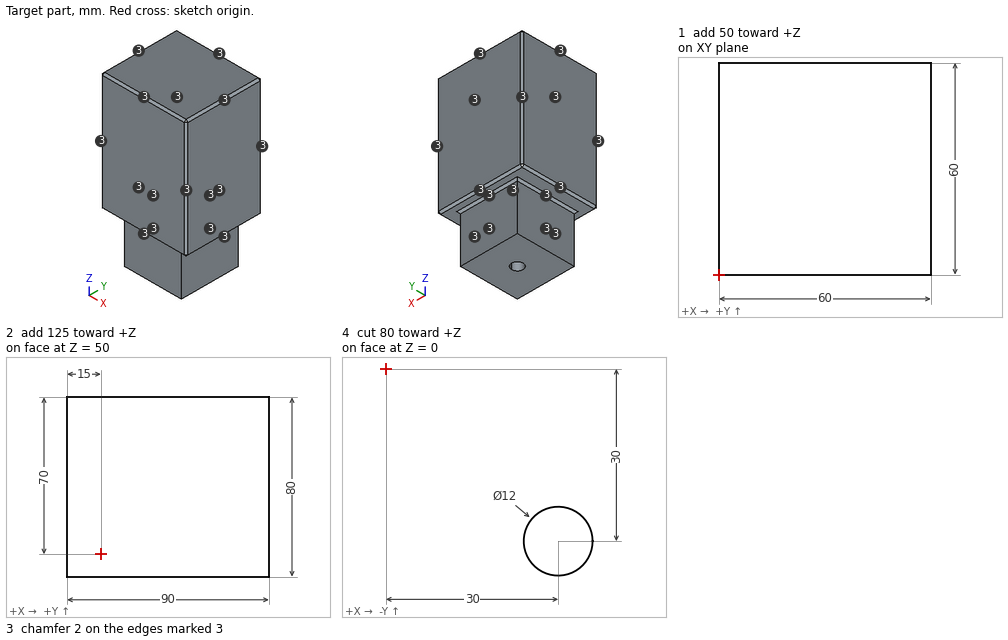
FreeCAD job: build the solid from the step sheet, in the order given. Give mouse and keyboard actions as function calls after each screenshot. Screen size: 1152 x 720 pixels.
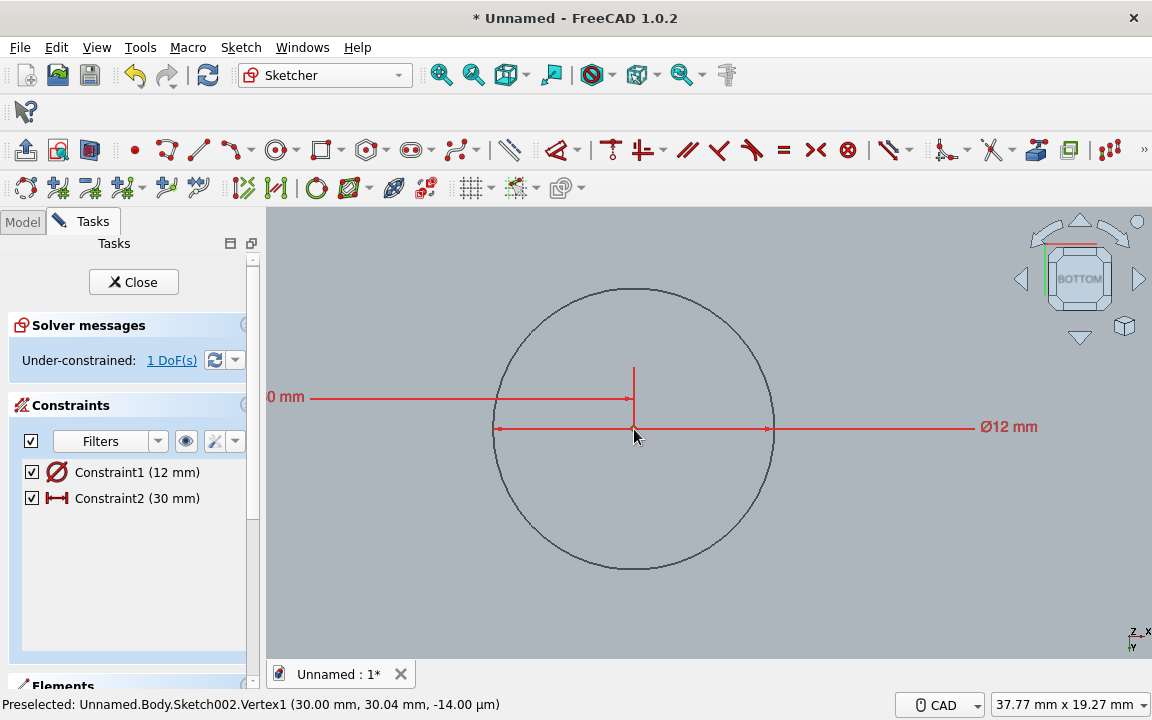
key(i)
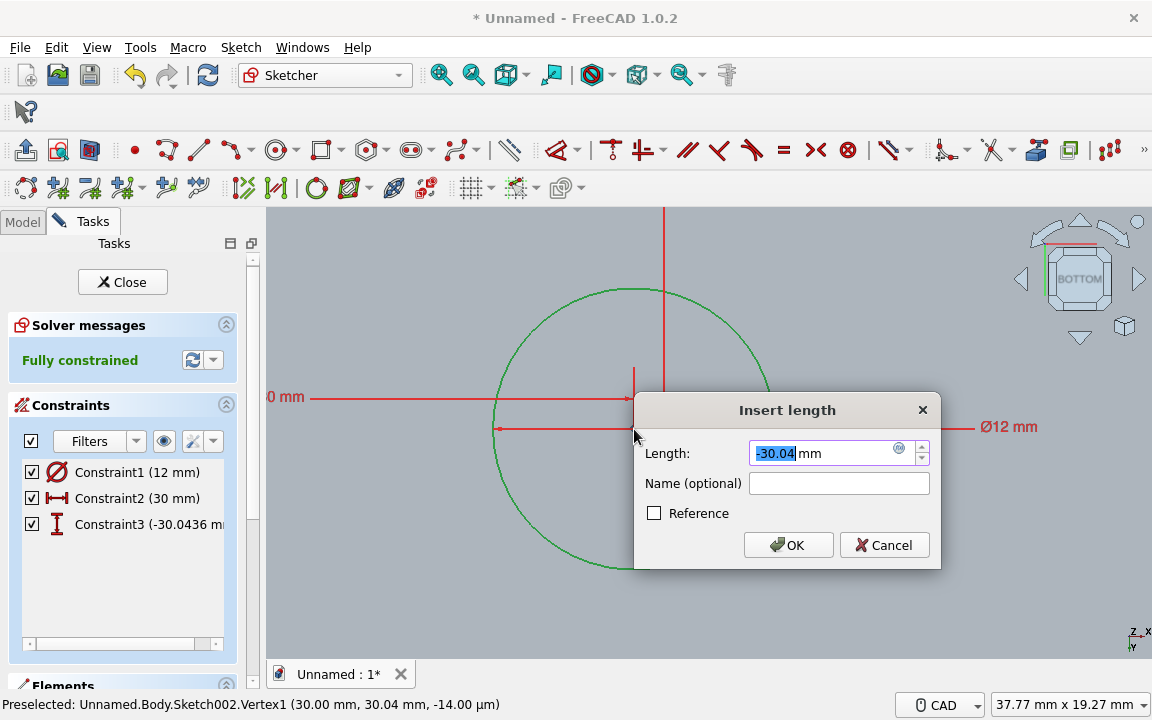
text(-30)
key(Return)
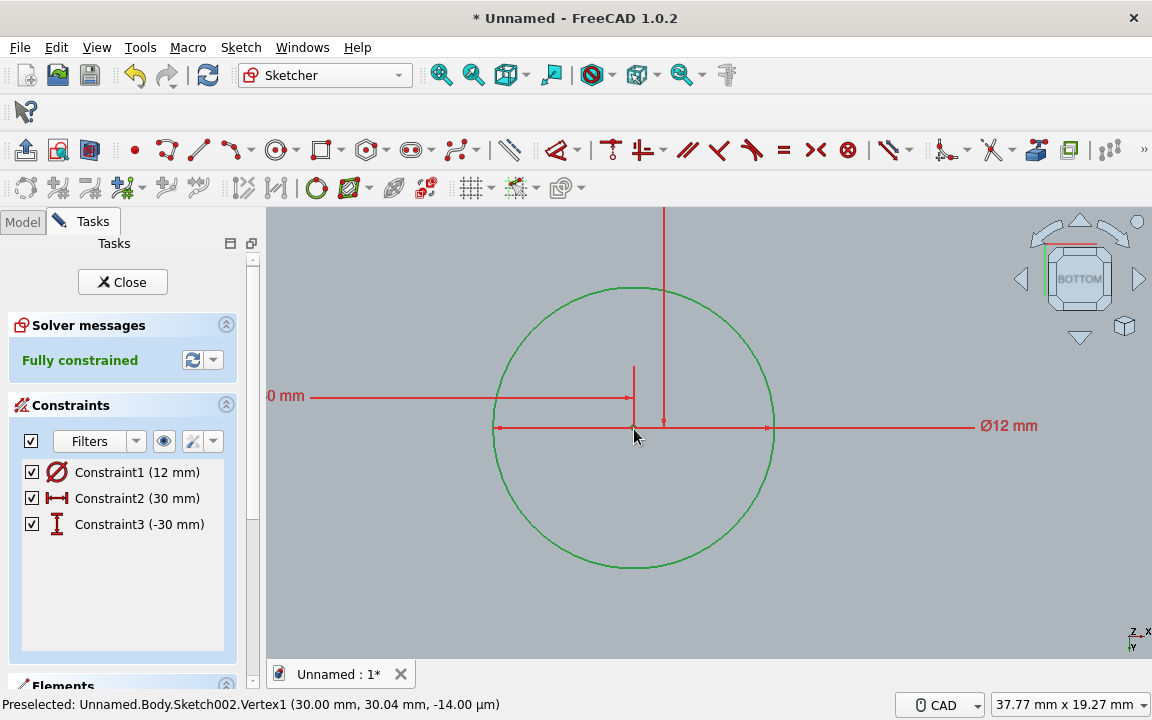
click(123, 282)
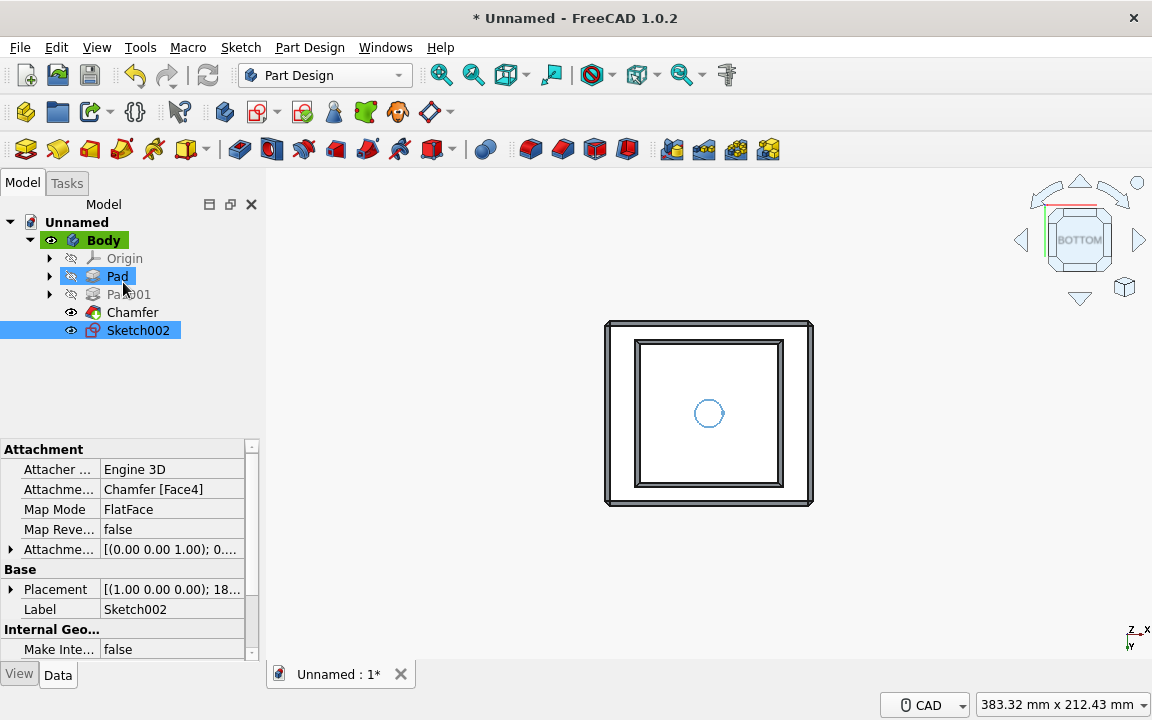
click(240, 150)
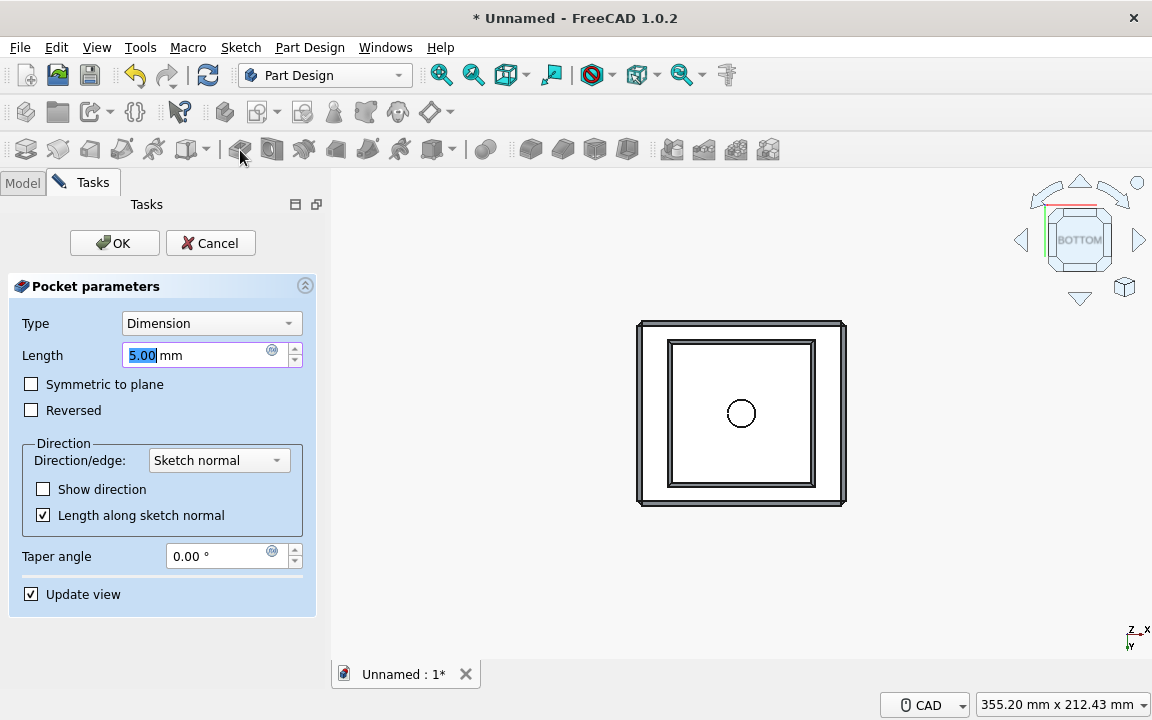
text(80)
key(Tab)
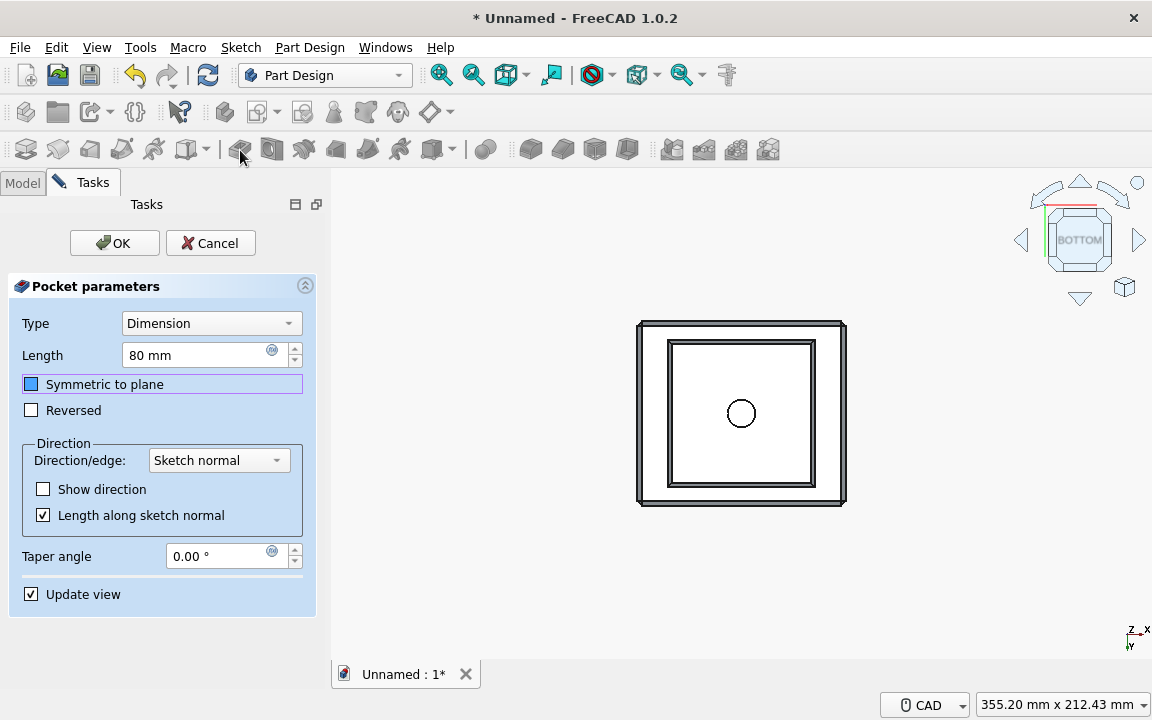
click(115, 243)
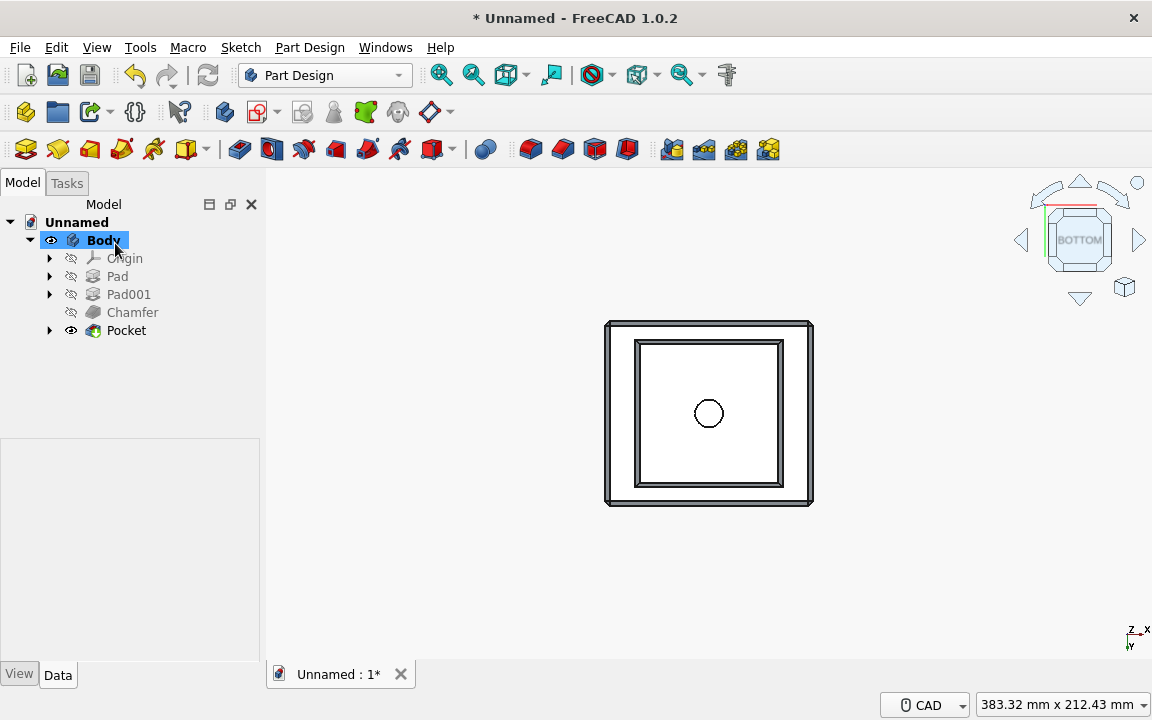
key(0)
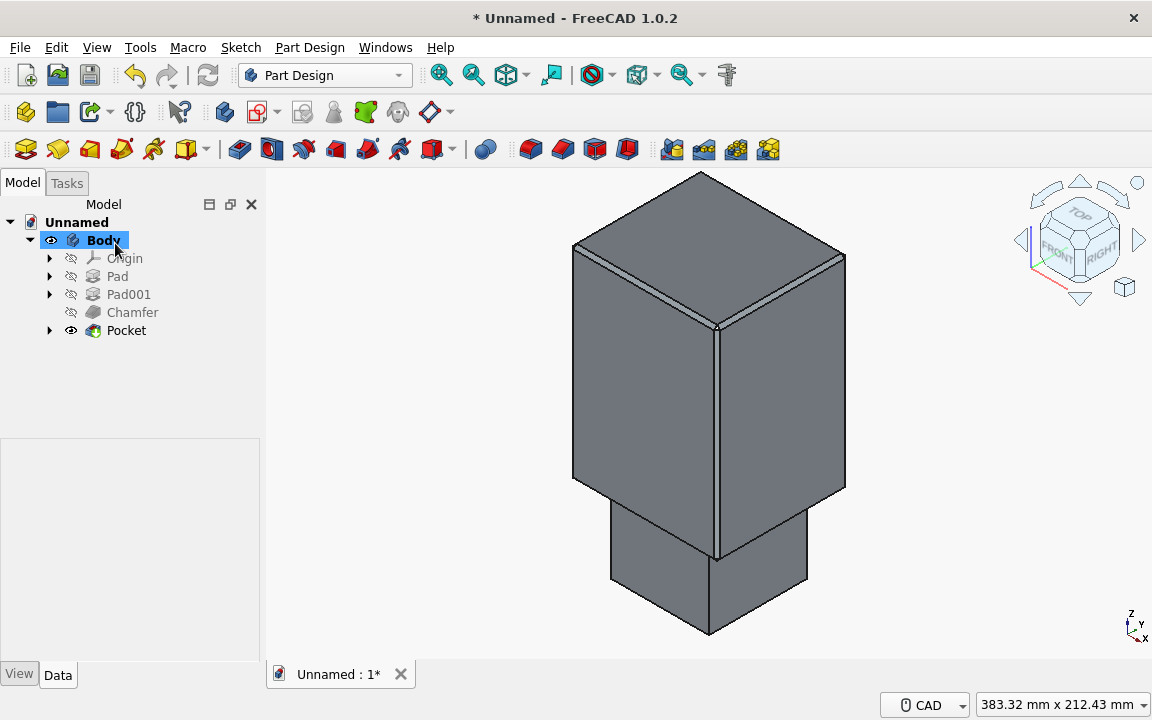
key(v)
key(f)